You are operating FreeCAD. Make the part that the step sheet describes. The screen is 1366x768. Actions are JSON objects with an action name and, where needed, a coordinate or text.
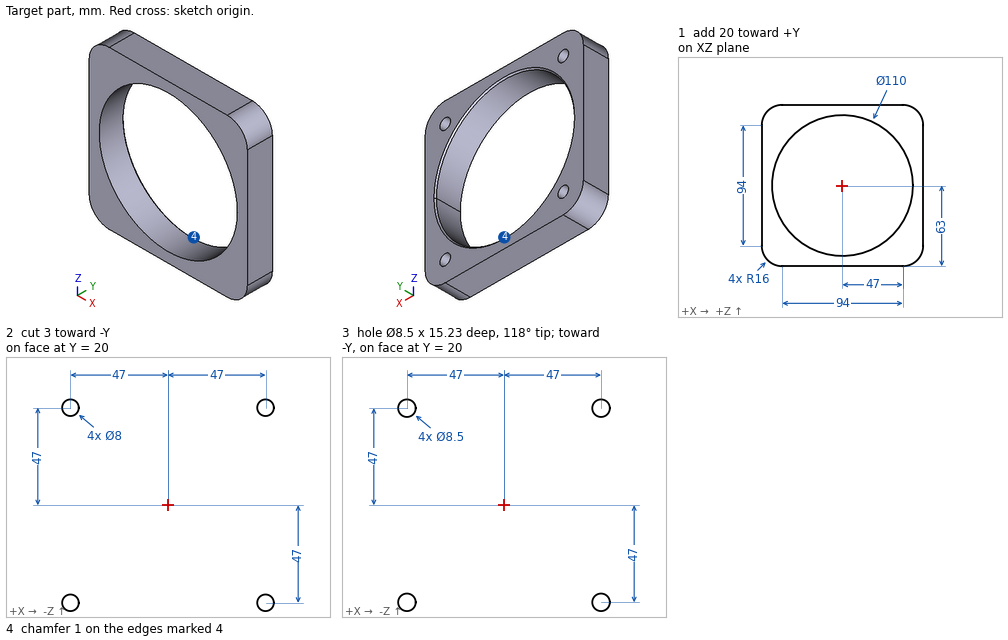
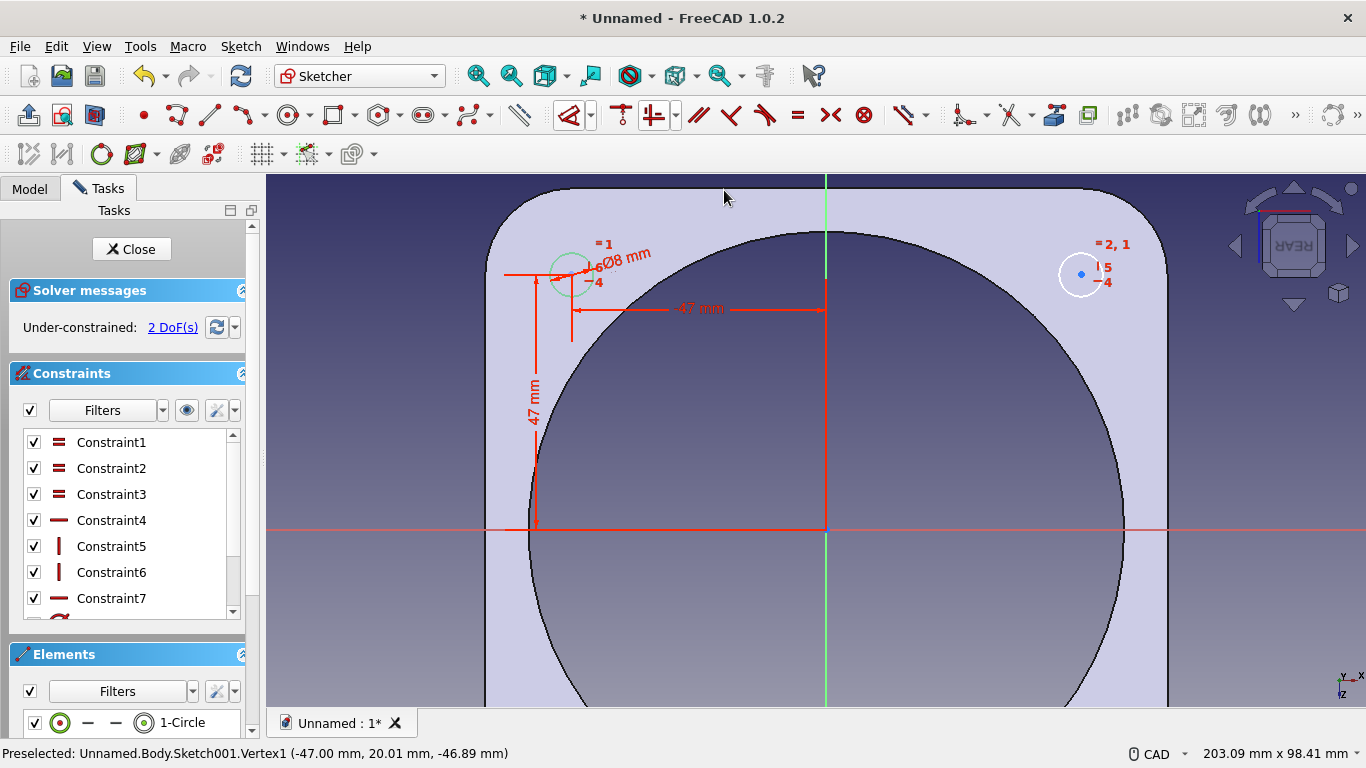
{"action": "left_click", "coordinate": [1081, 275]}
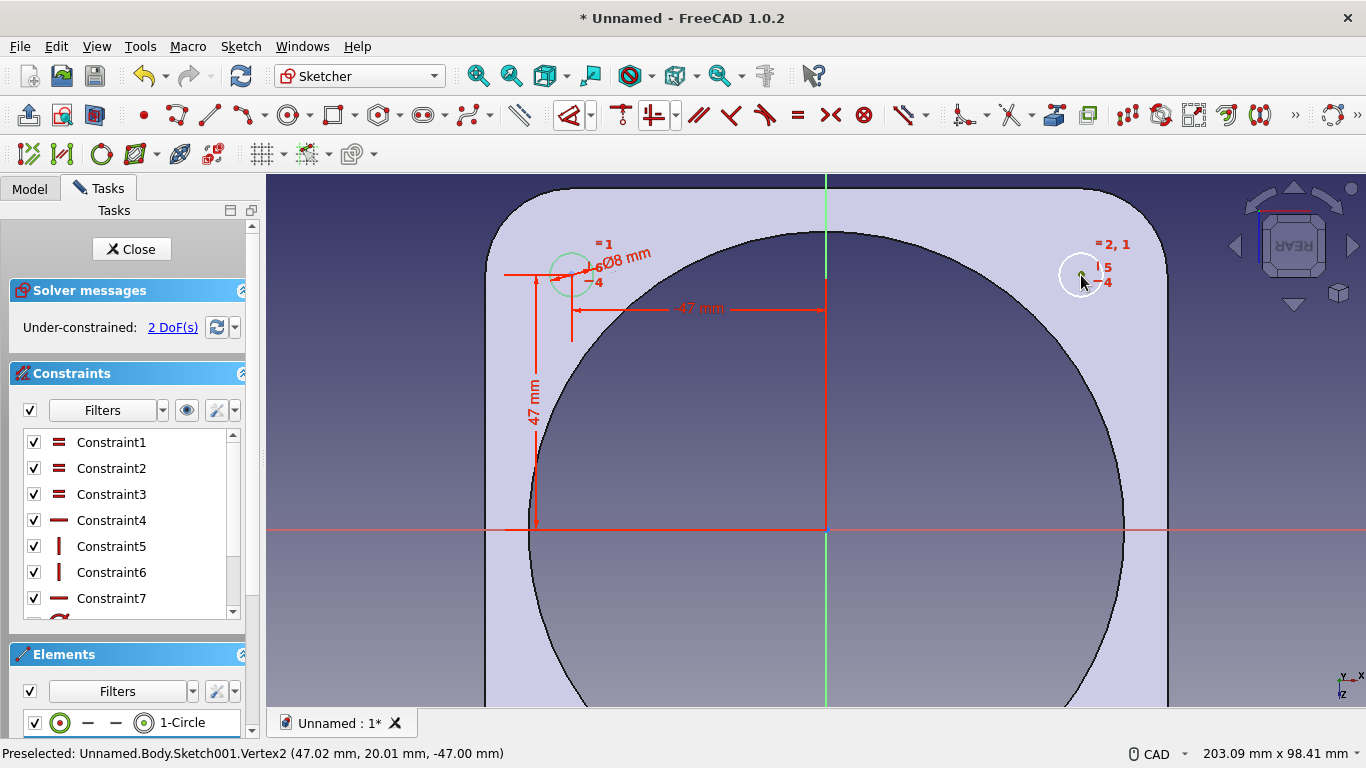
{"action": "left_click", "coordinate": [590, 116]}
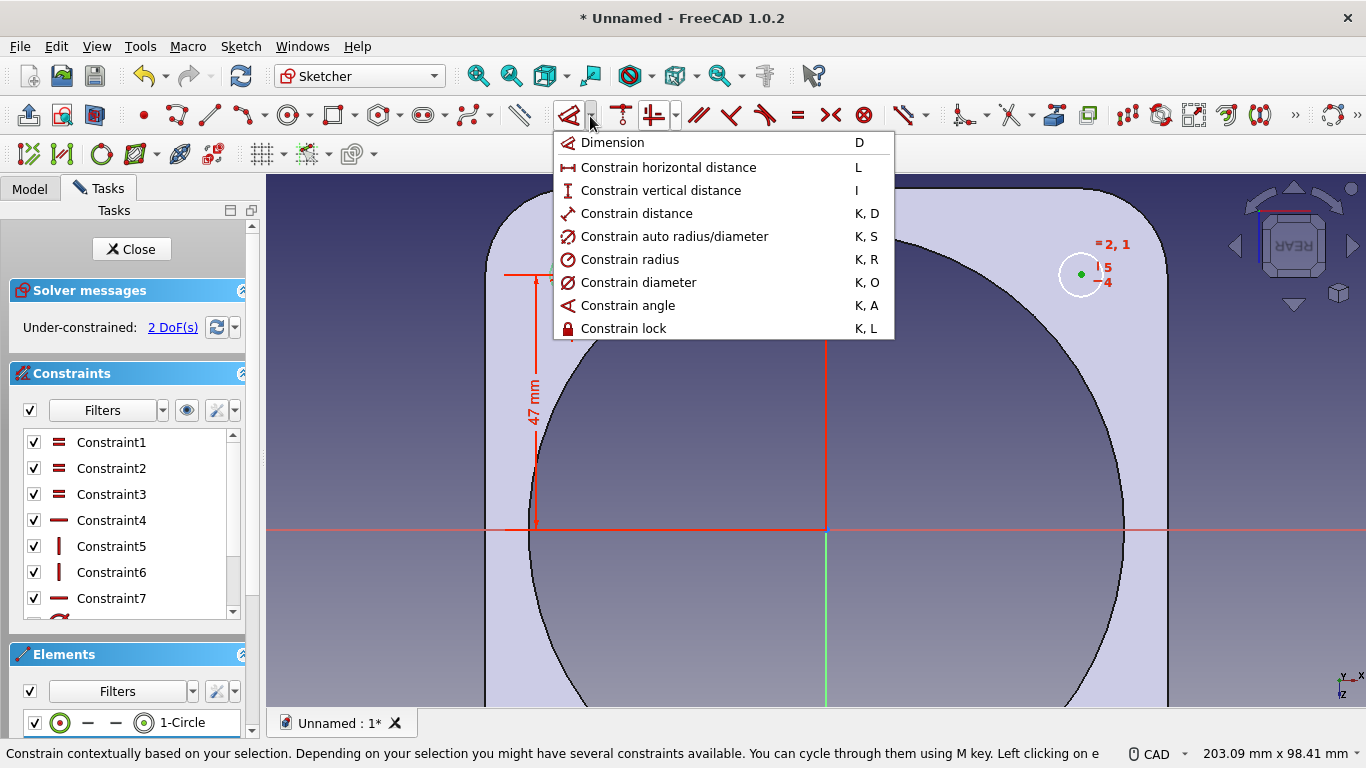
{"action": "left_click", "coordinate": [724, 168]}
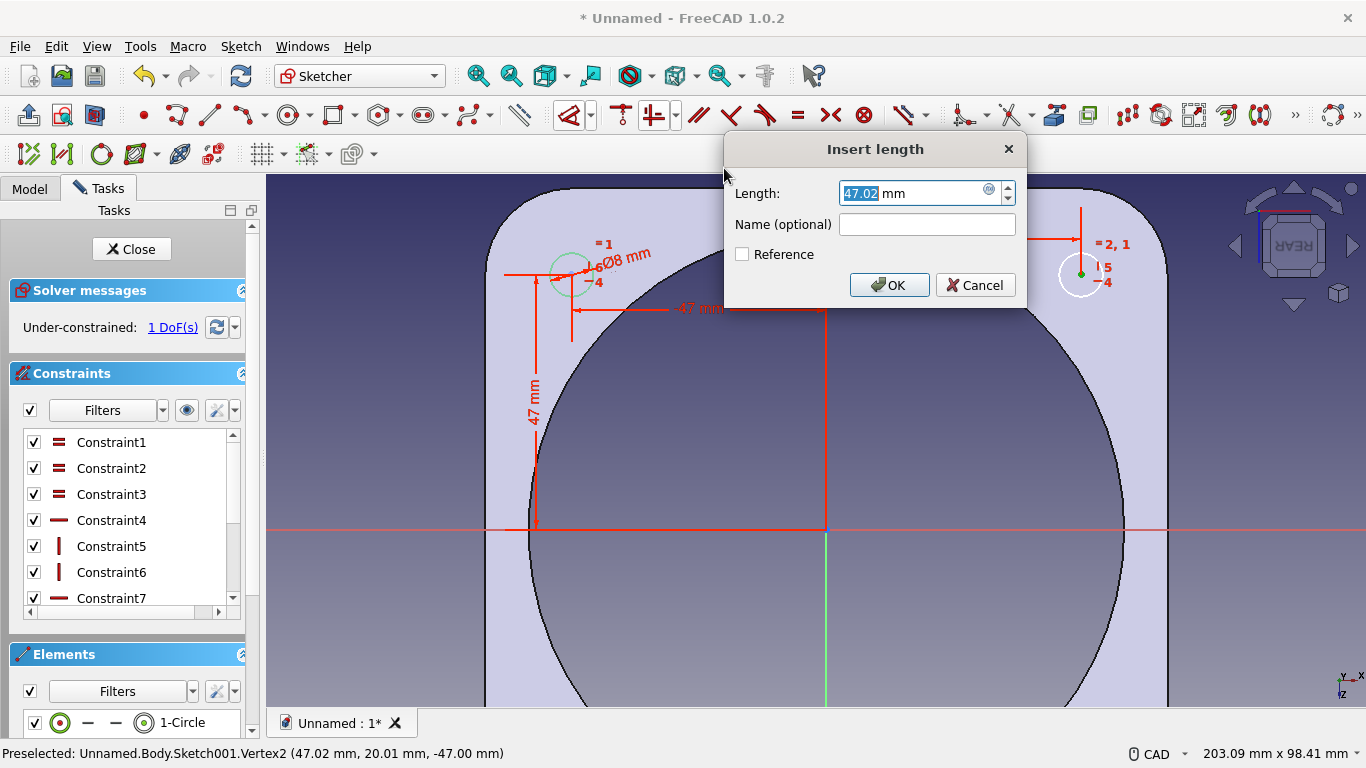
{"action": "type", "text": "47"}
{"action": "key", "text": "Return"}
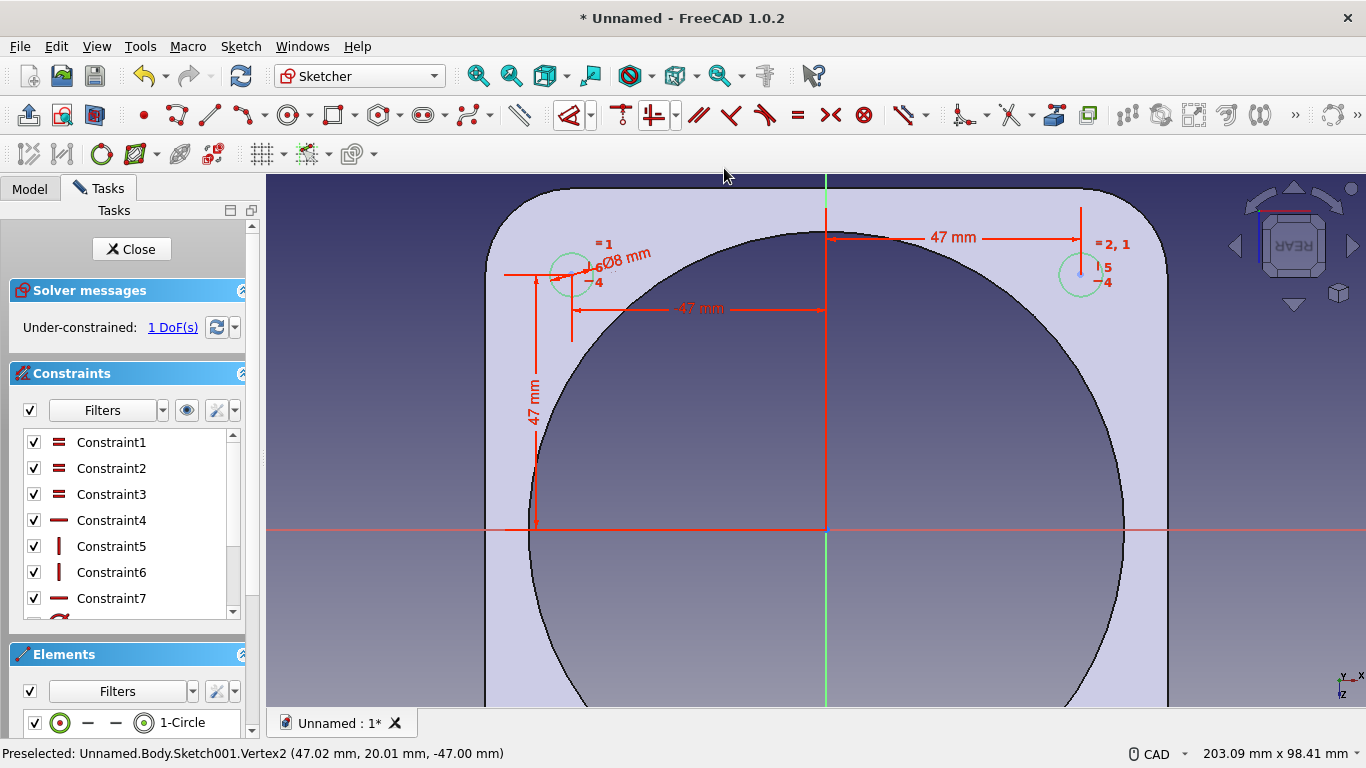
{"action": "scroll", "coordinate": [587, 260], "scroll_direction": "down", "scroll_amount": 2}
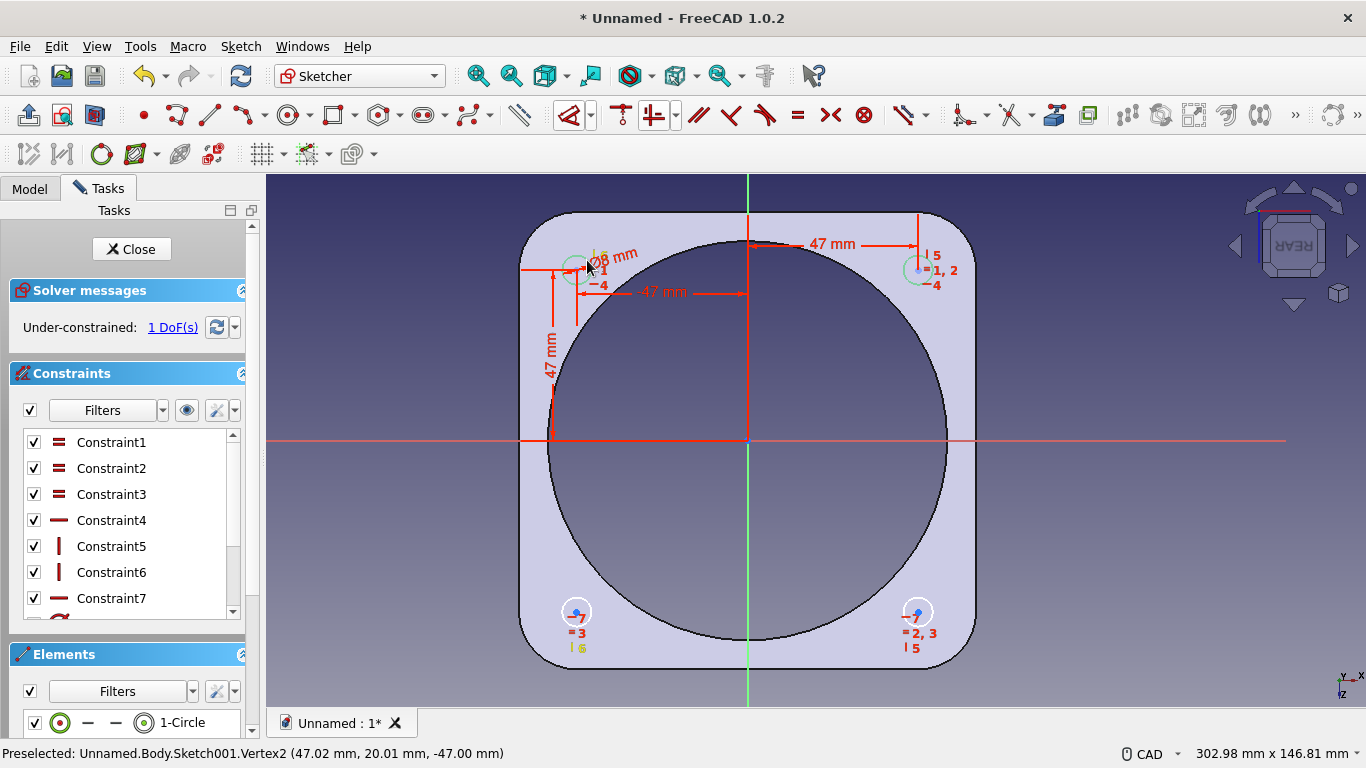
{"action": "left_click", "coordinate": [918, 612]}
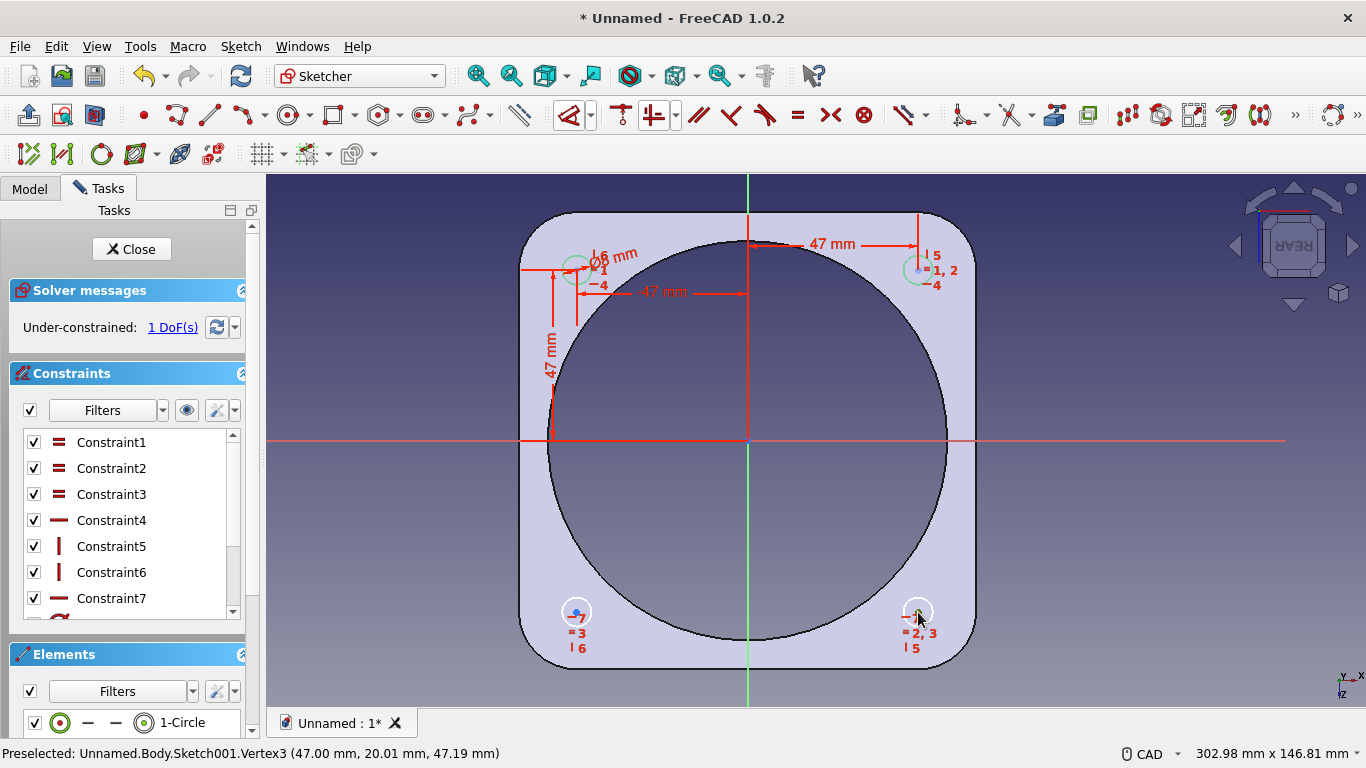
{"action": "key", "text": "i"}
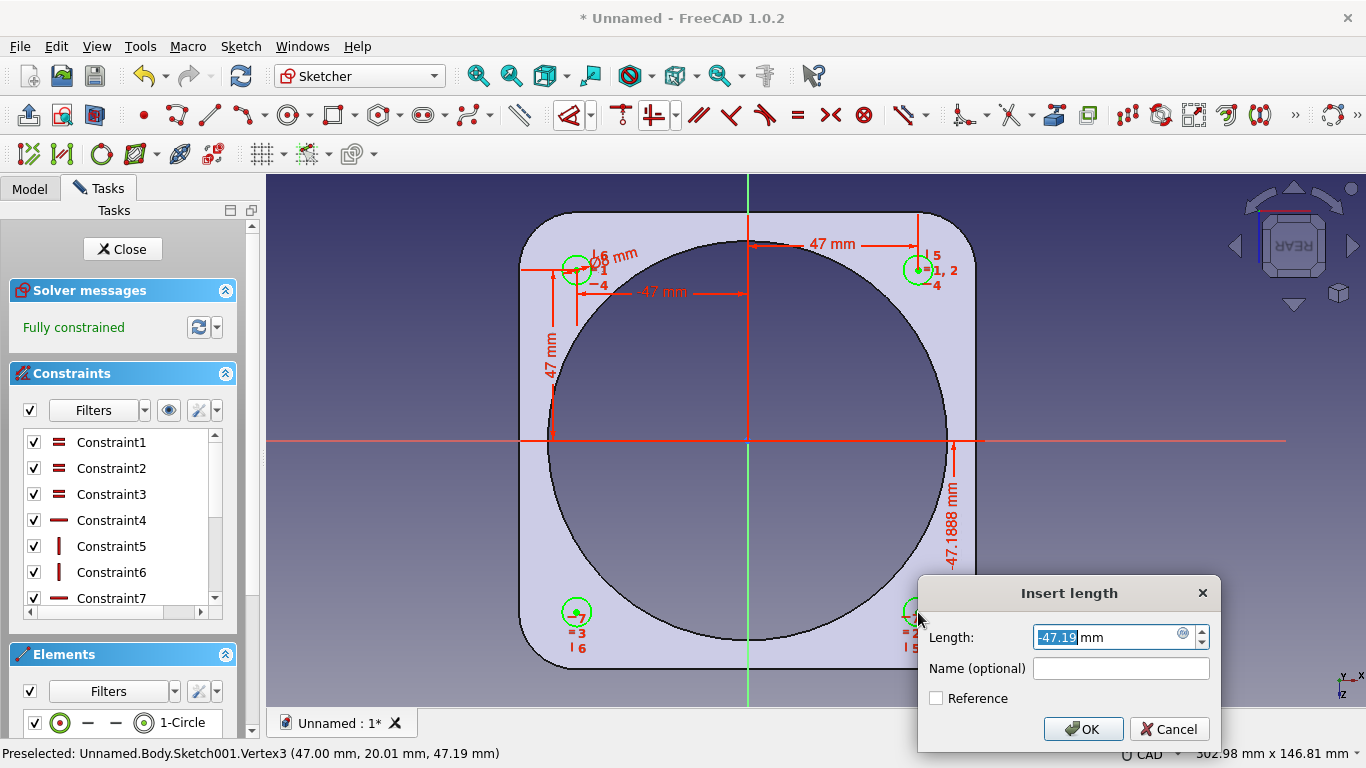
{"action": "type", "text": "-47"}
{"action": "key", "text": "Return"}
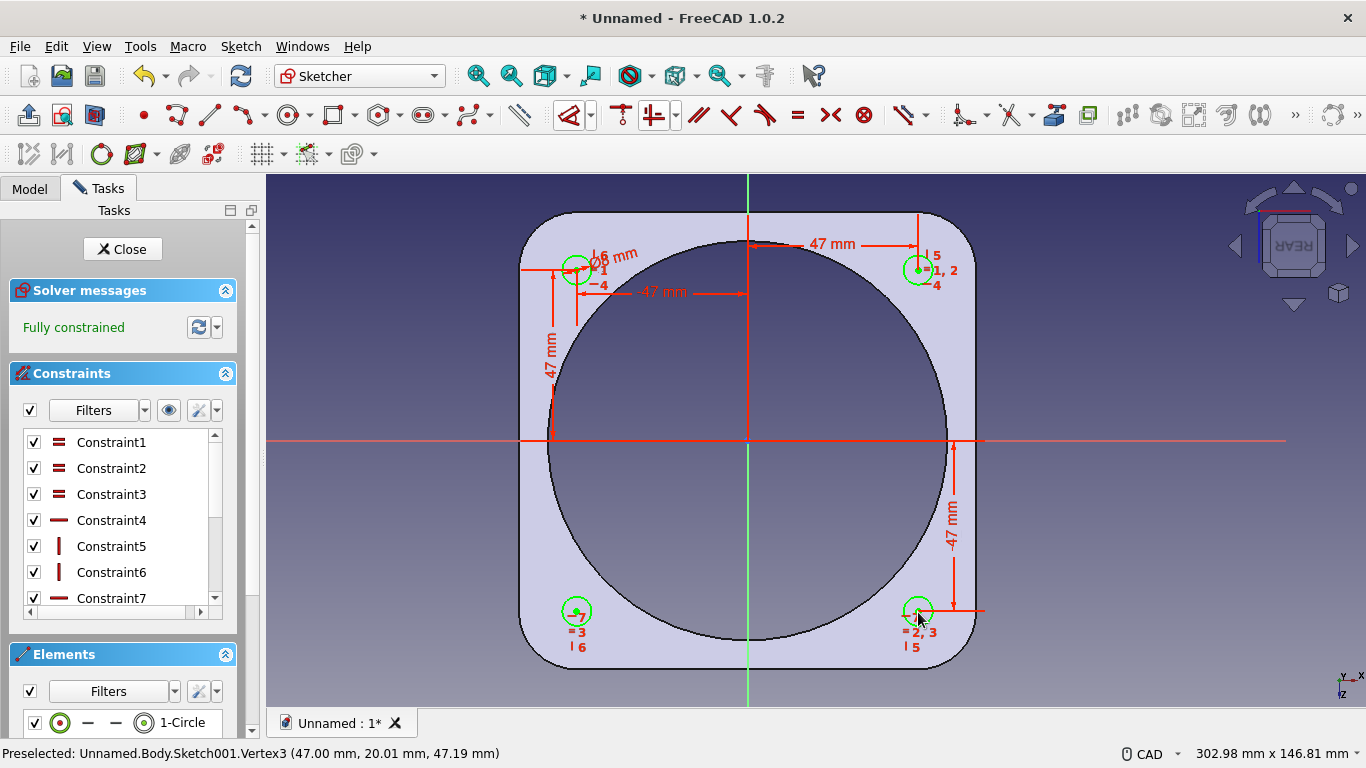
{"action": "left_click", "coordinate": [123, 249]}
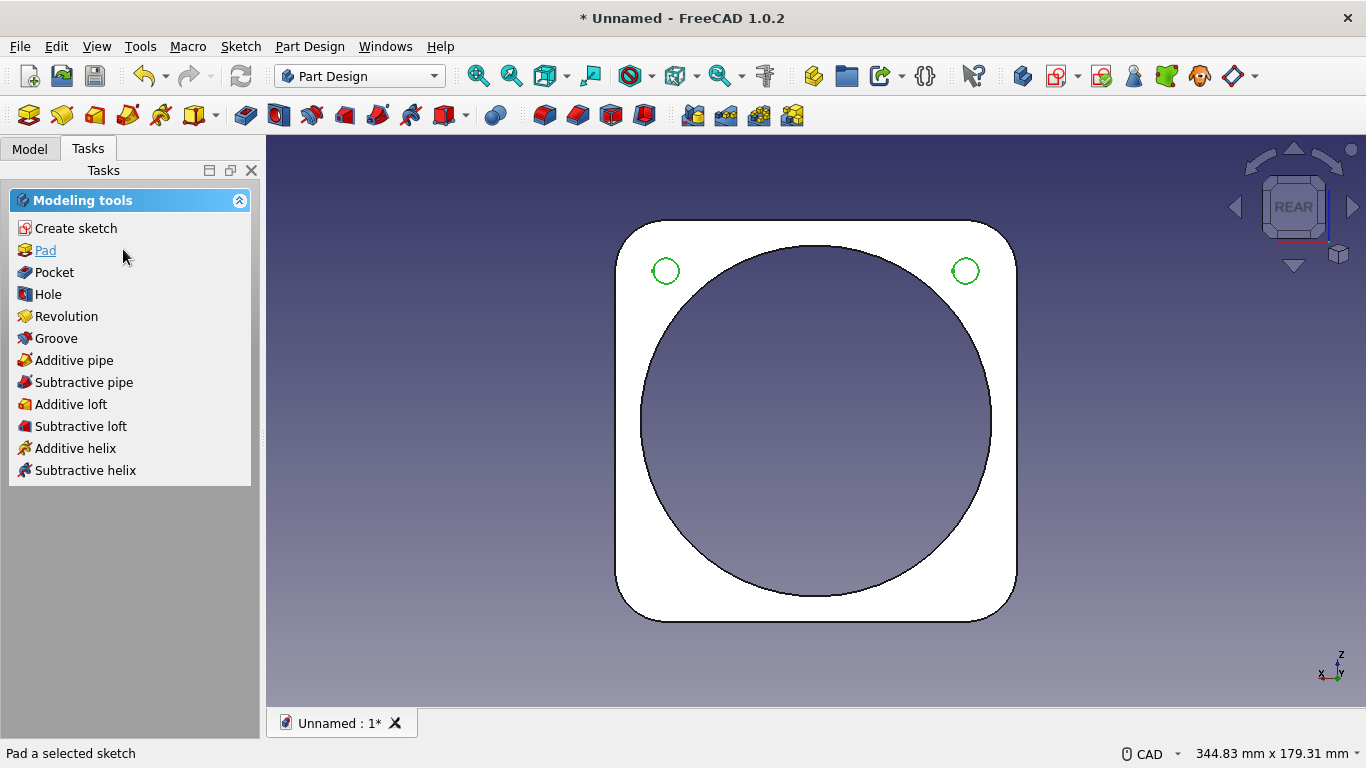
{"action": "left_click", "coordinate": [246, 116]}